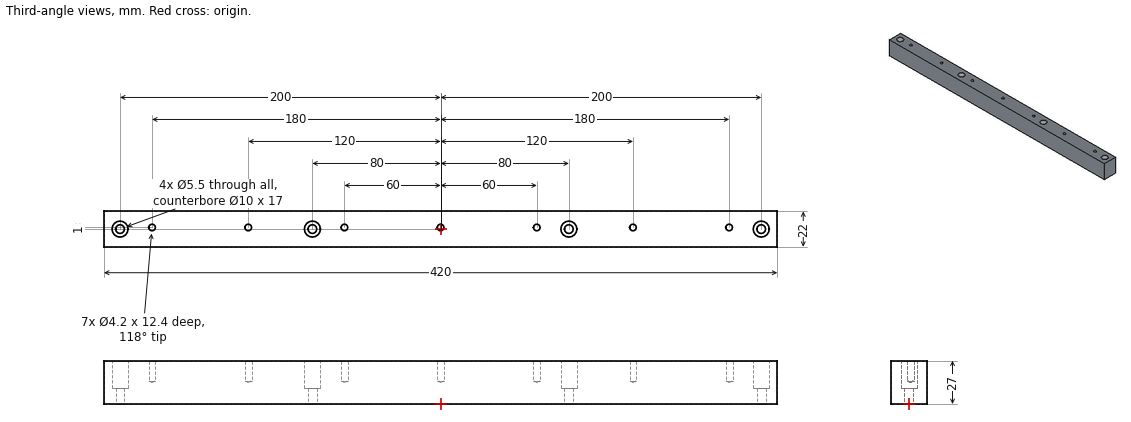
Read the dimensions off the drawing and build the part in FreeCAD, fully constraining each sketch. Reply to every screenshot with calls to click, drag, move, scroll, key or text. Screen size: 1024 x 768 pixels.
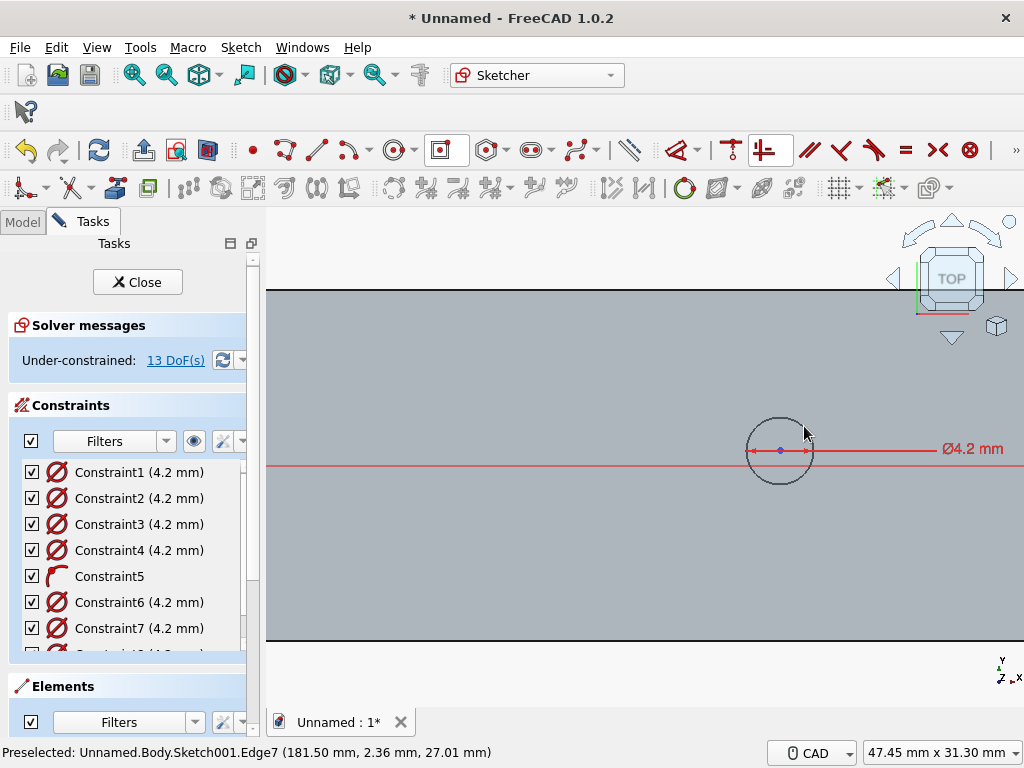
scroll(791, 458, down, 13)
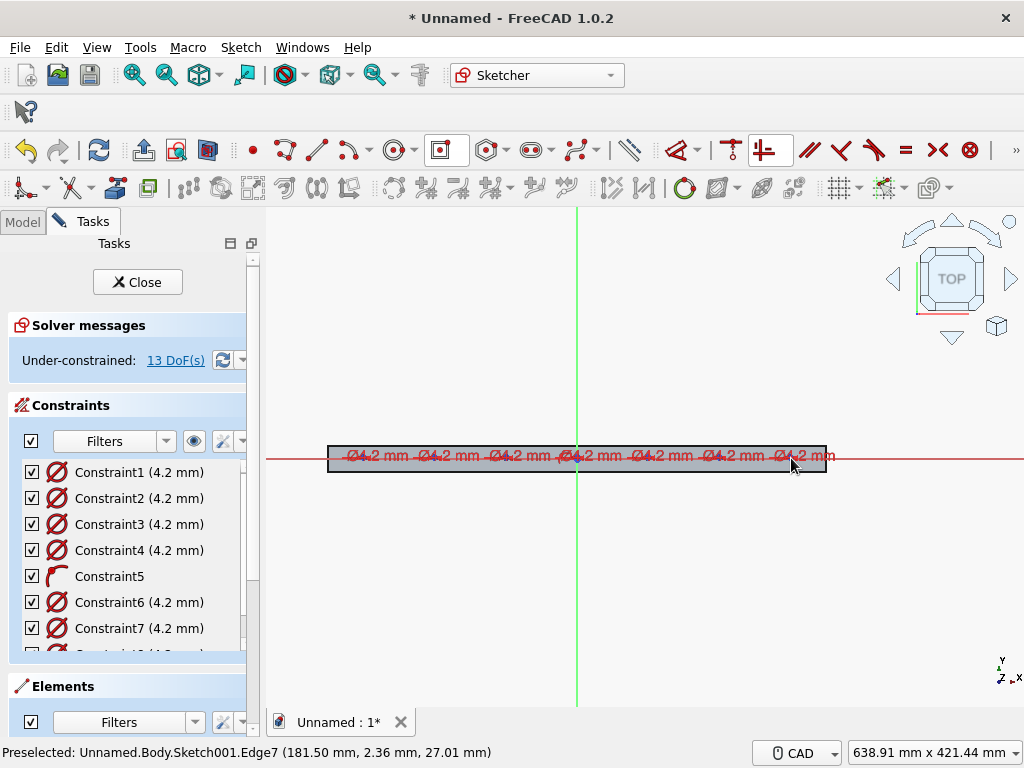
click(364, 458)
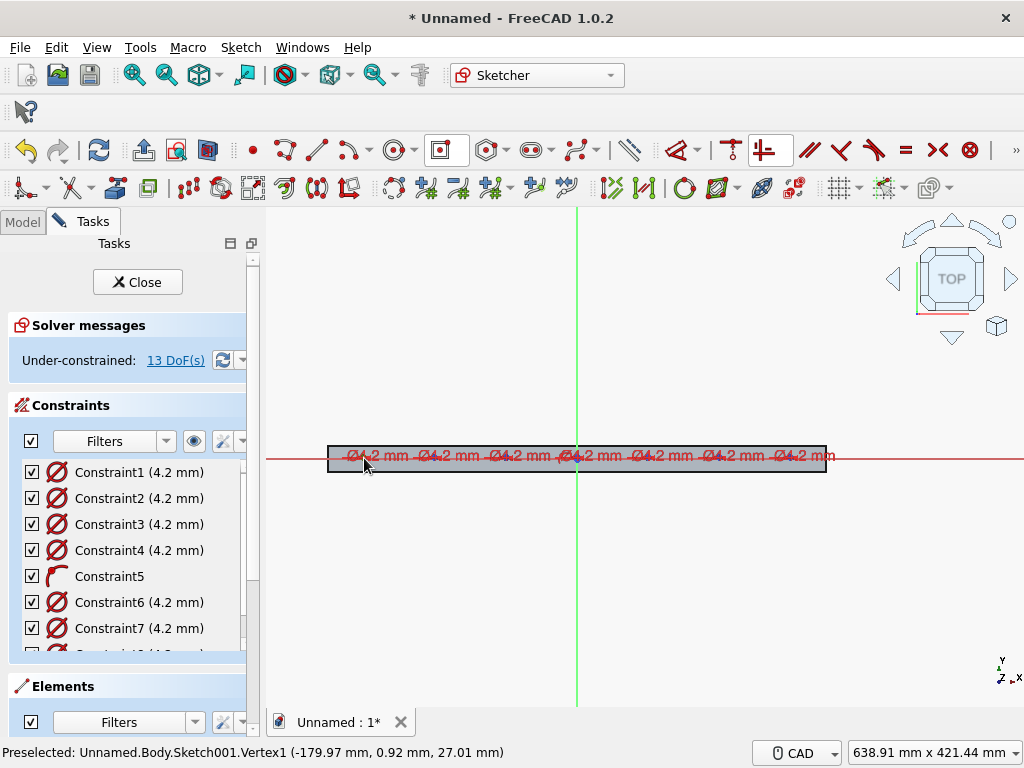
click(435, 458)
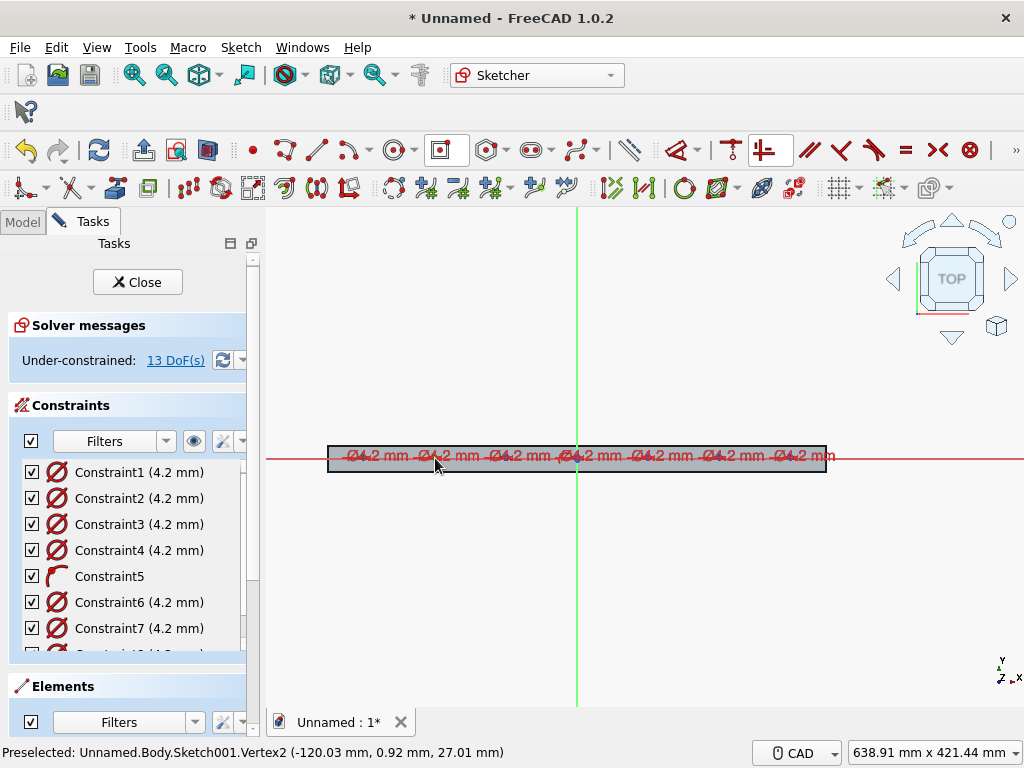
key(h)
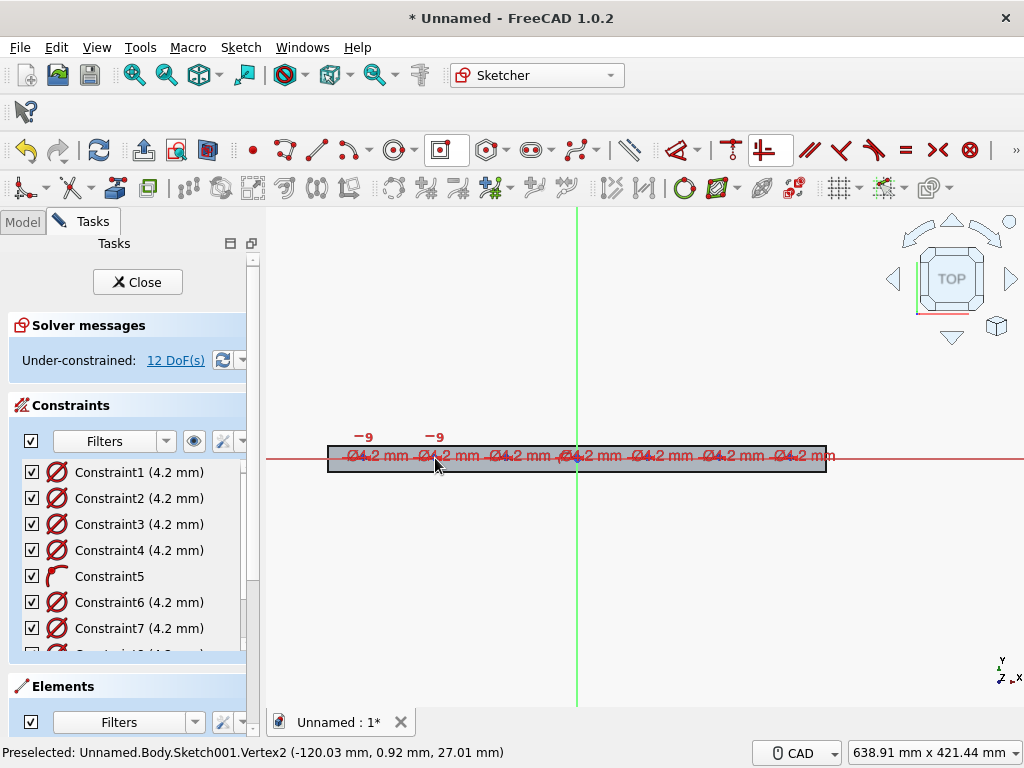
click(435, 458)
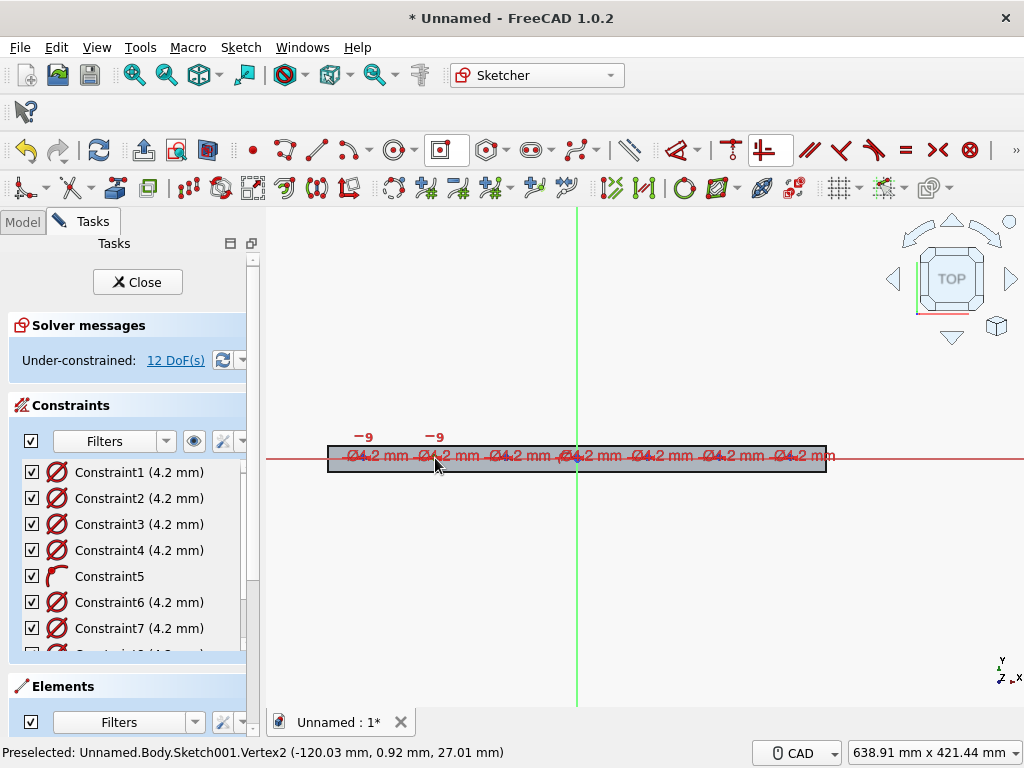
click(506, 458)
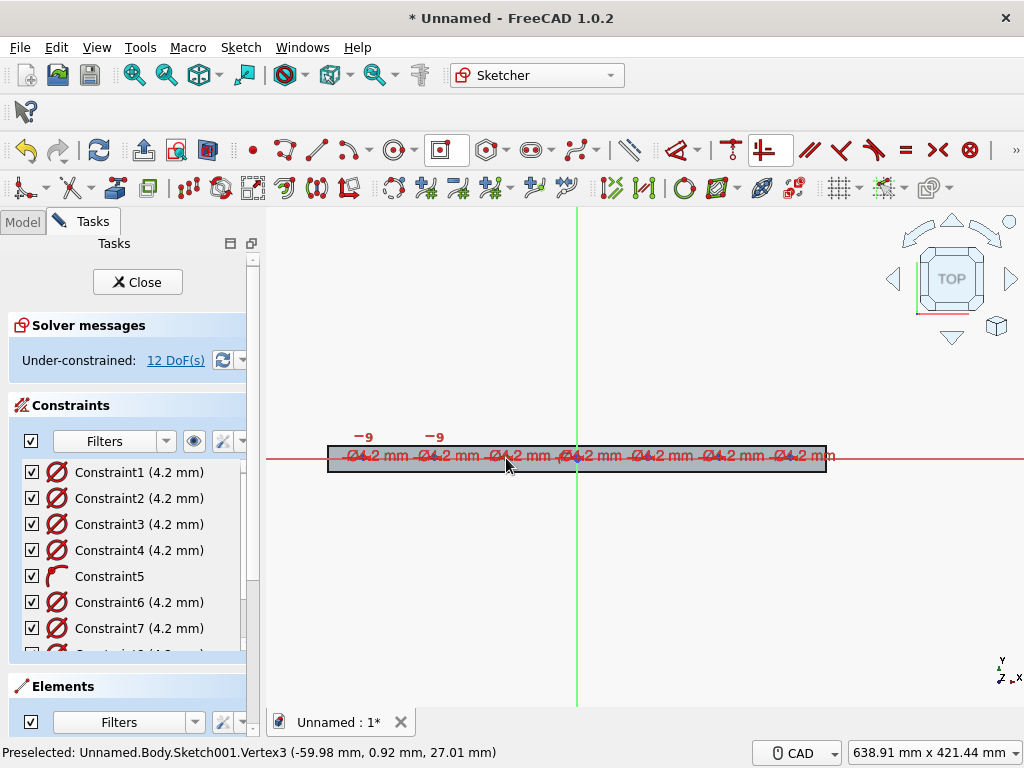
key(h)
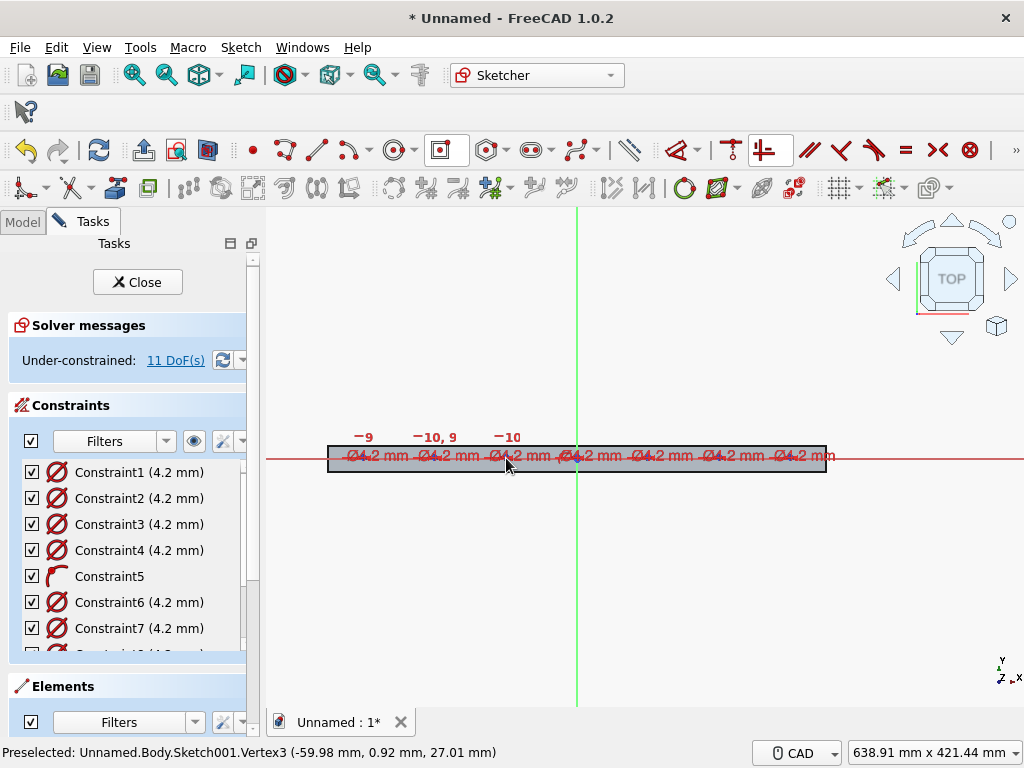
click(506, 458)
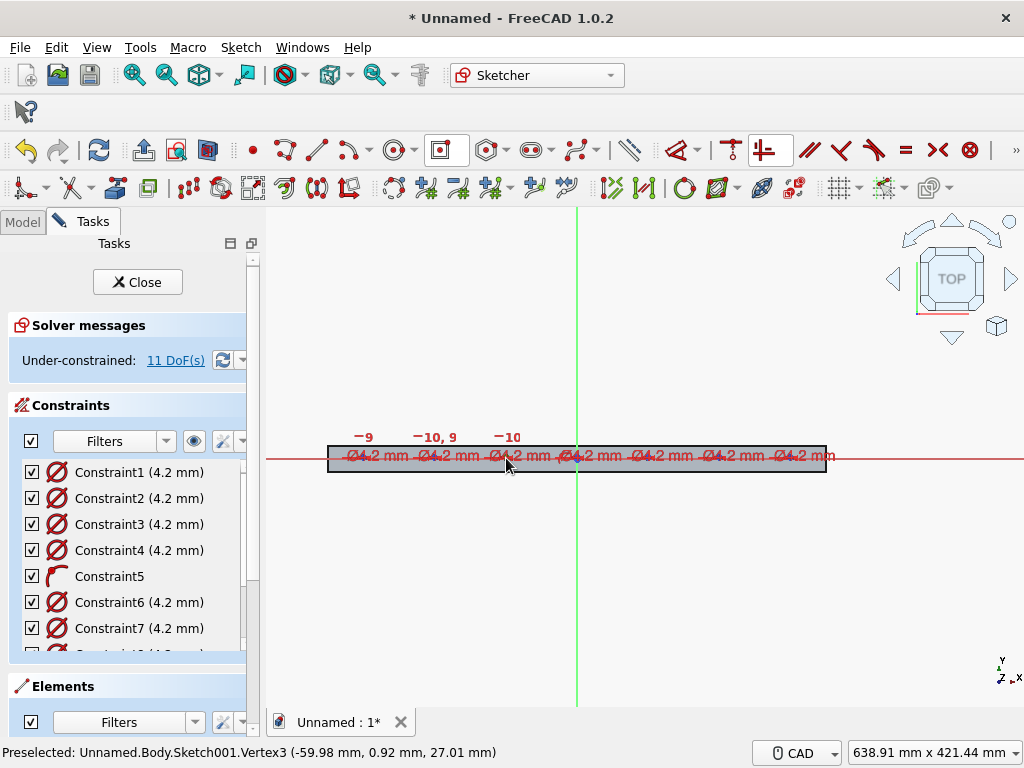
scroll(577, 458, up, 13)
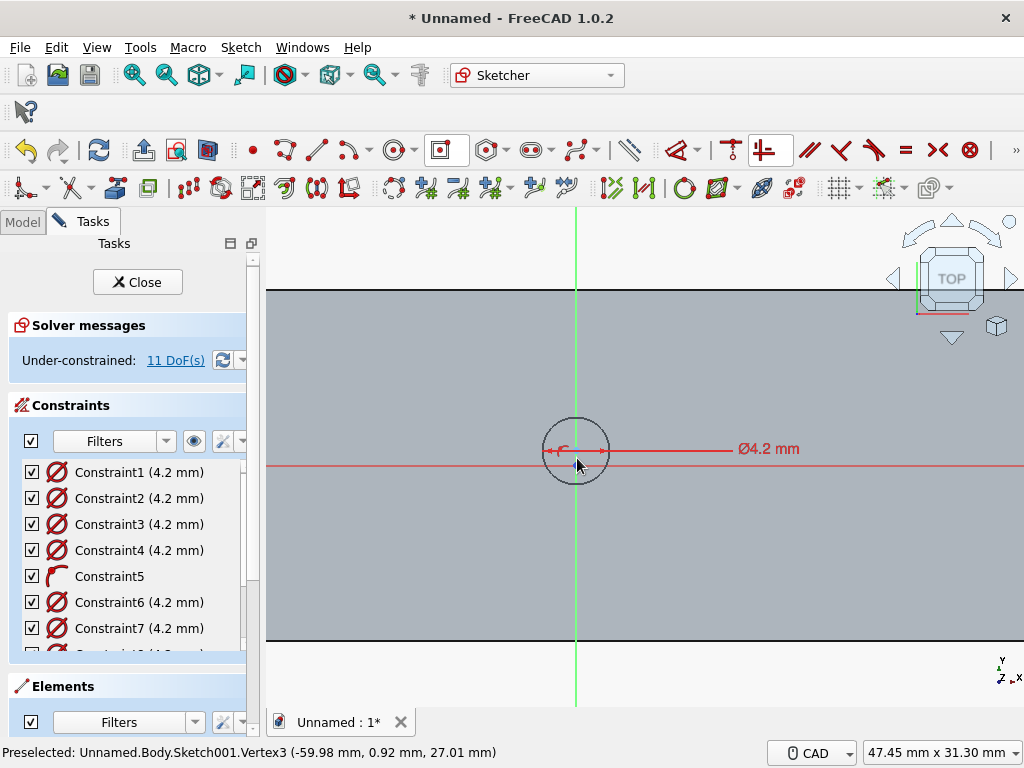
click(576, 451)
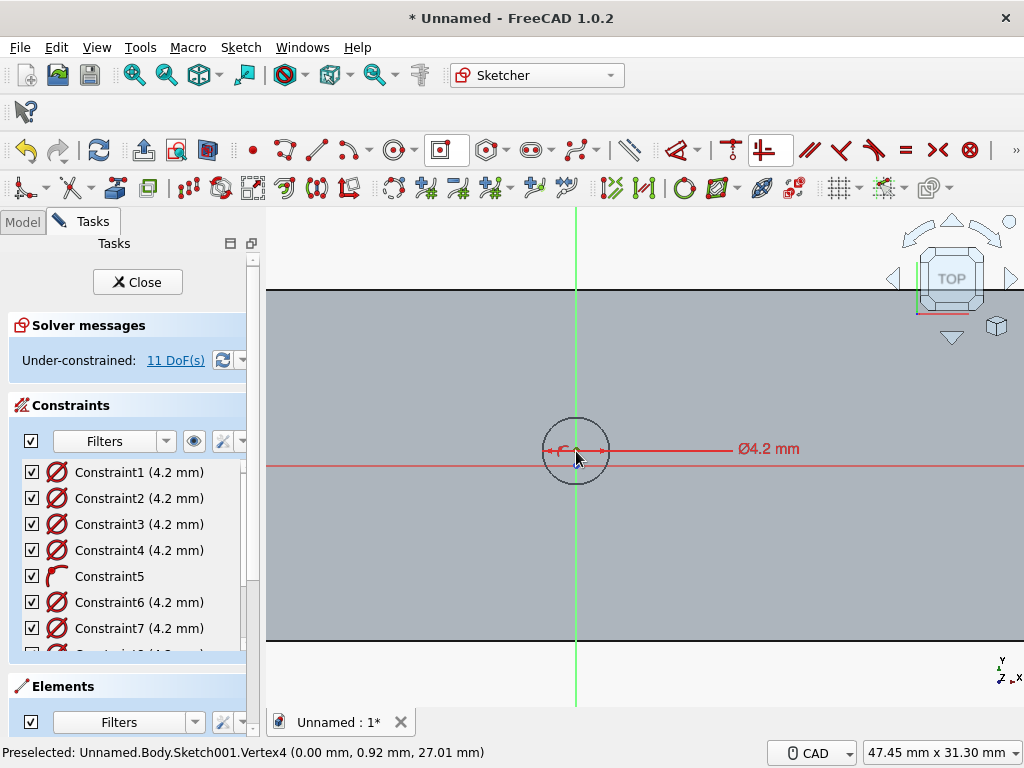
key(h)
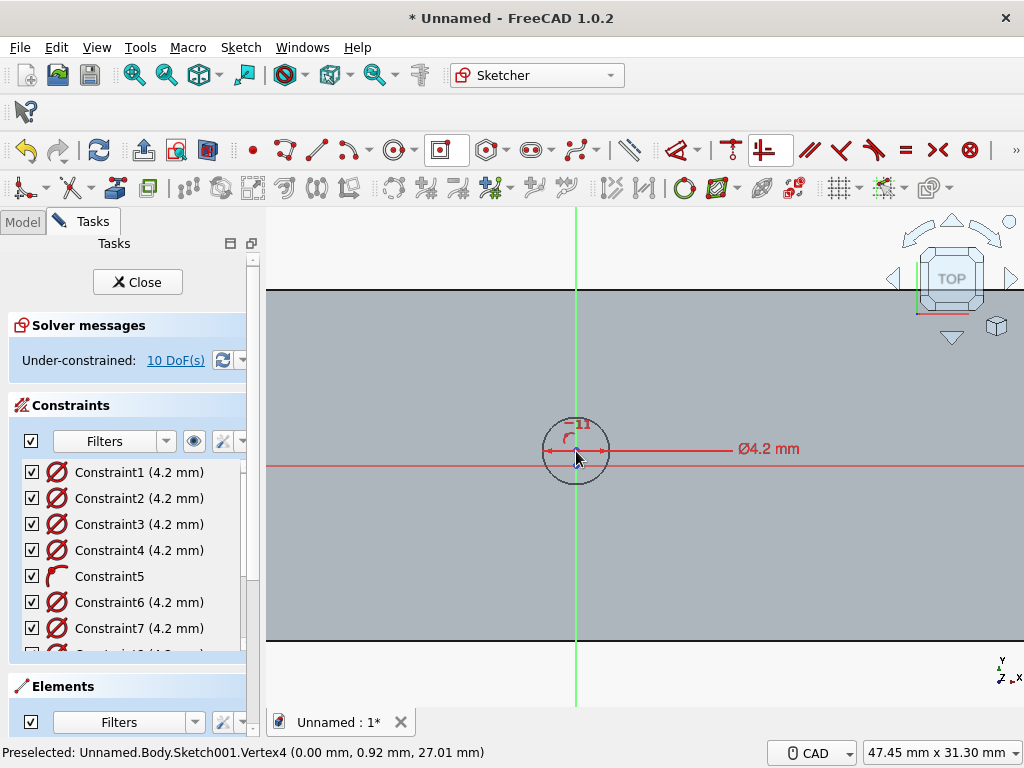
click(576, 451)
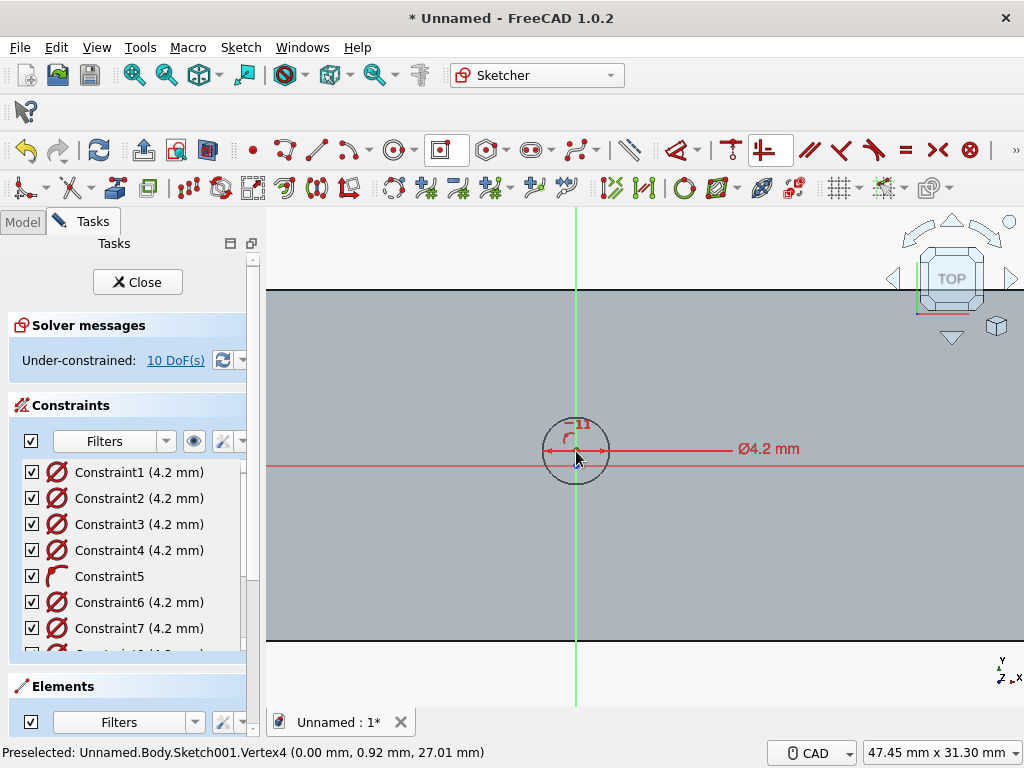
scroll(577, 458, down, 13)